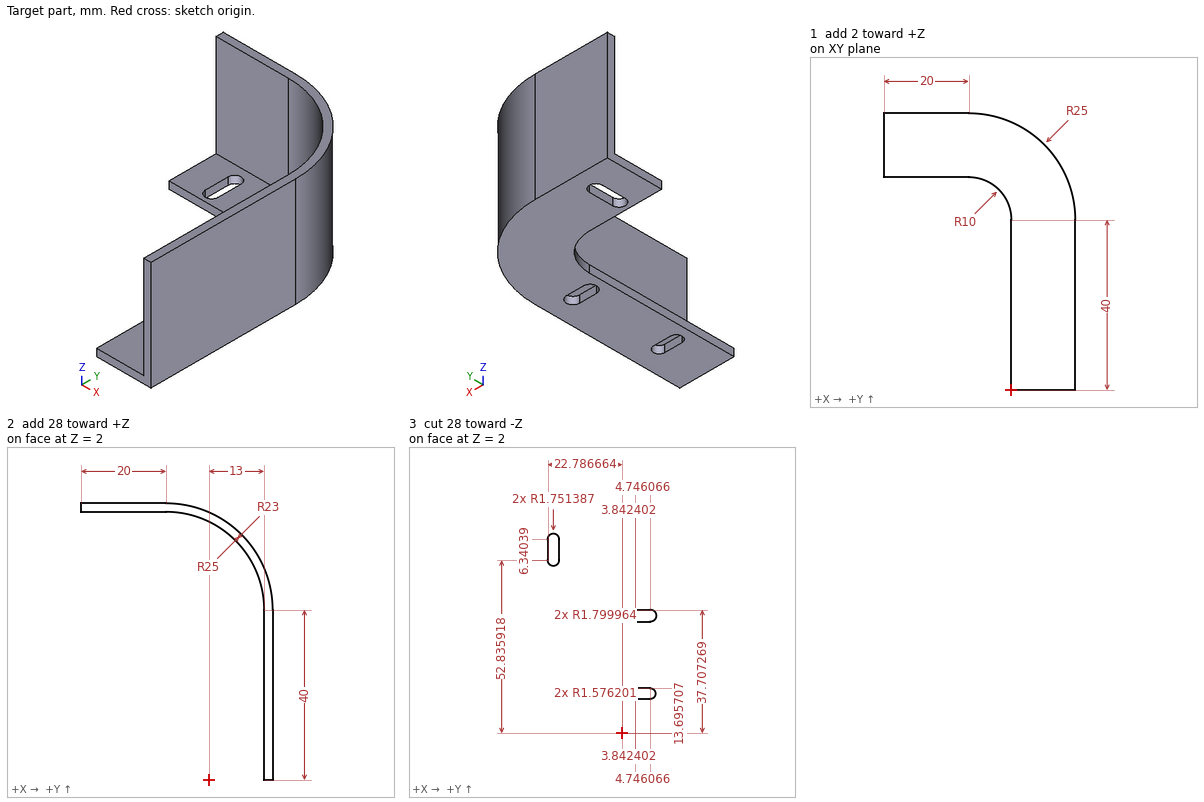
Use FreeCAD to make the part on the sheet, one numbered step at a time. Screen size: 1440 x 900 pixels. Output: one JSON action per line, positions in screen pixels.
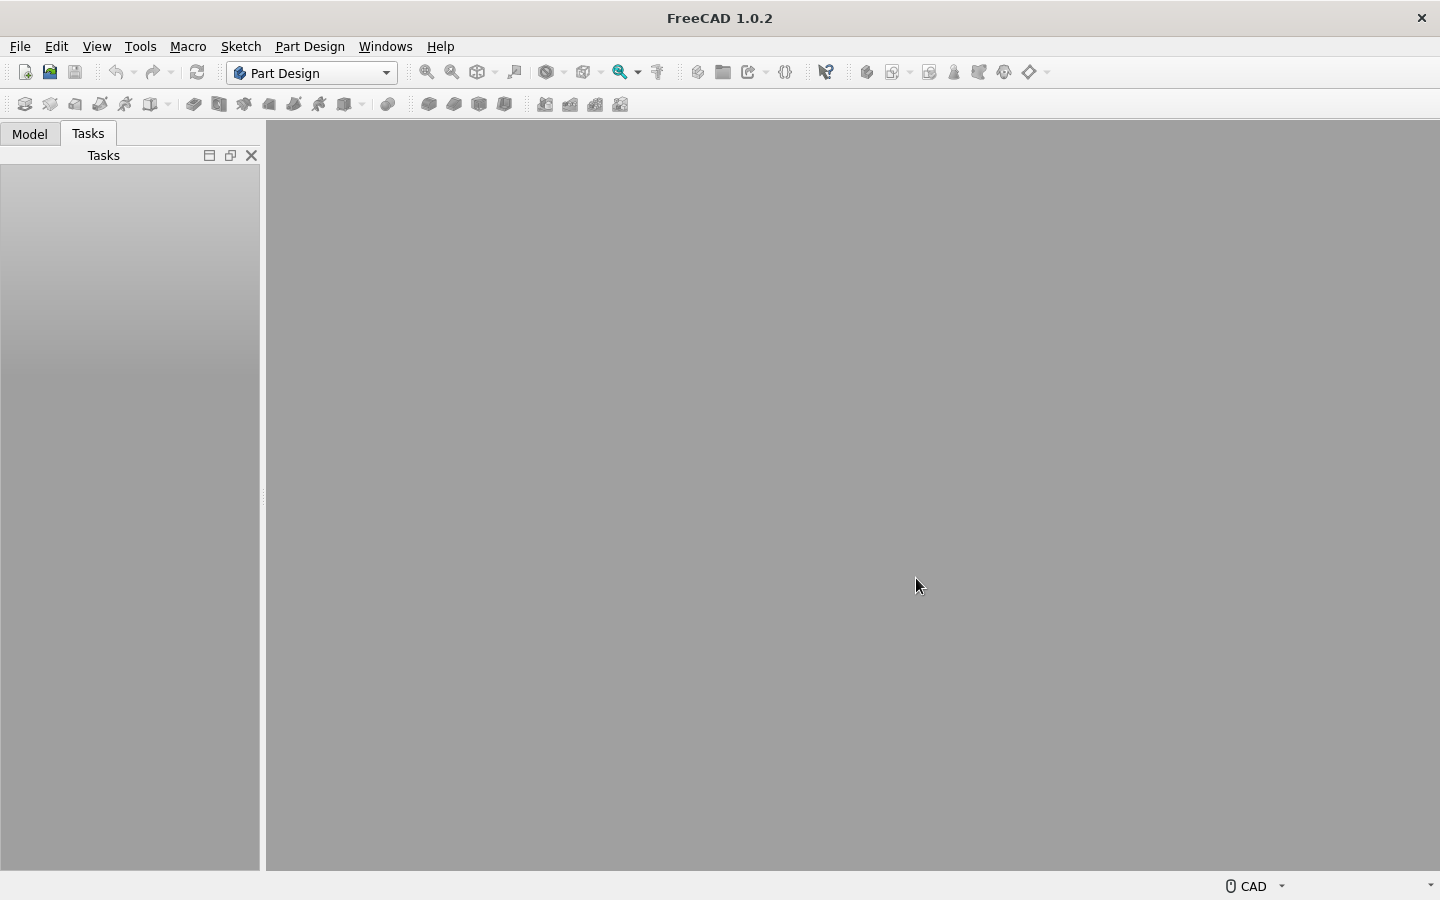
{"action": "left_click", "coordinate": [25, 72]}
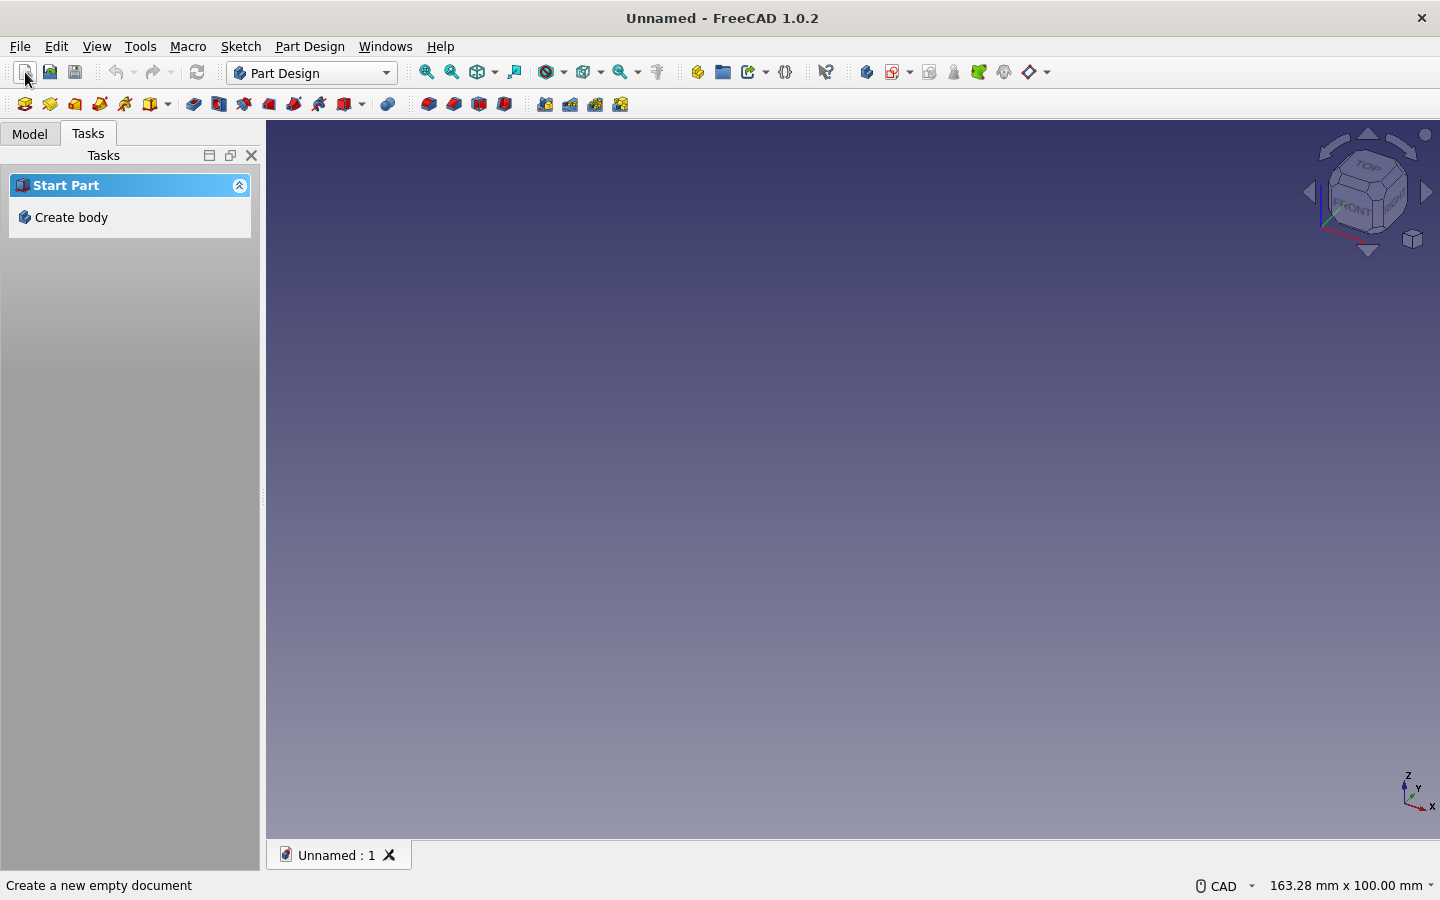
{"action": "left_click", "coordinate": [892, 72]}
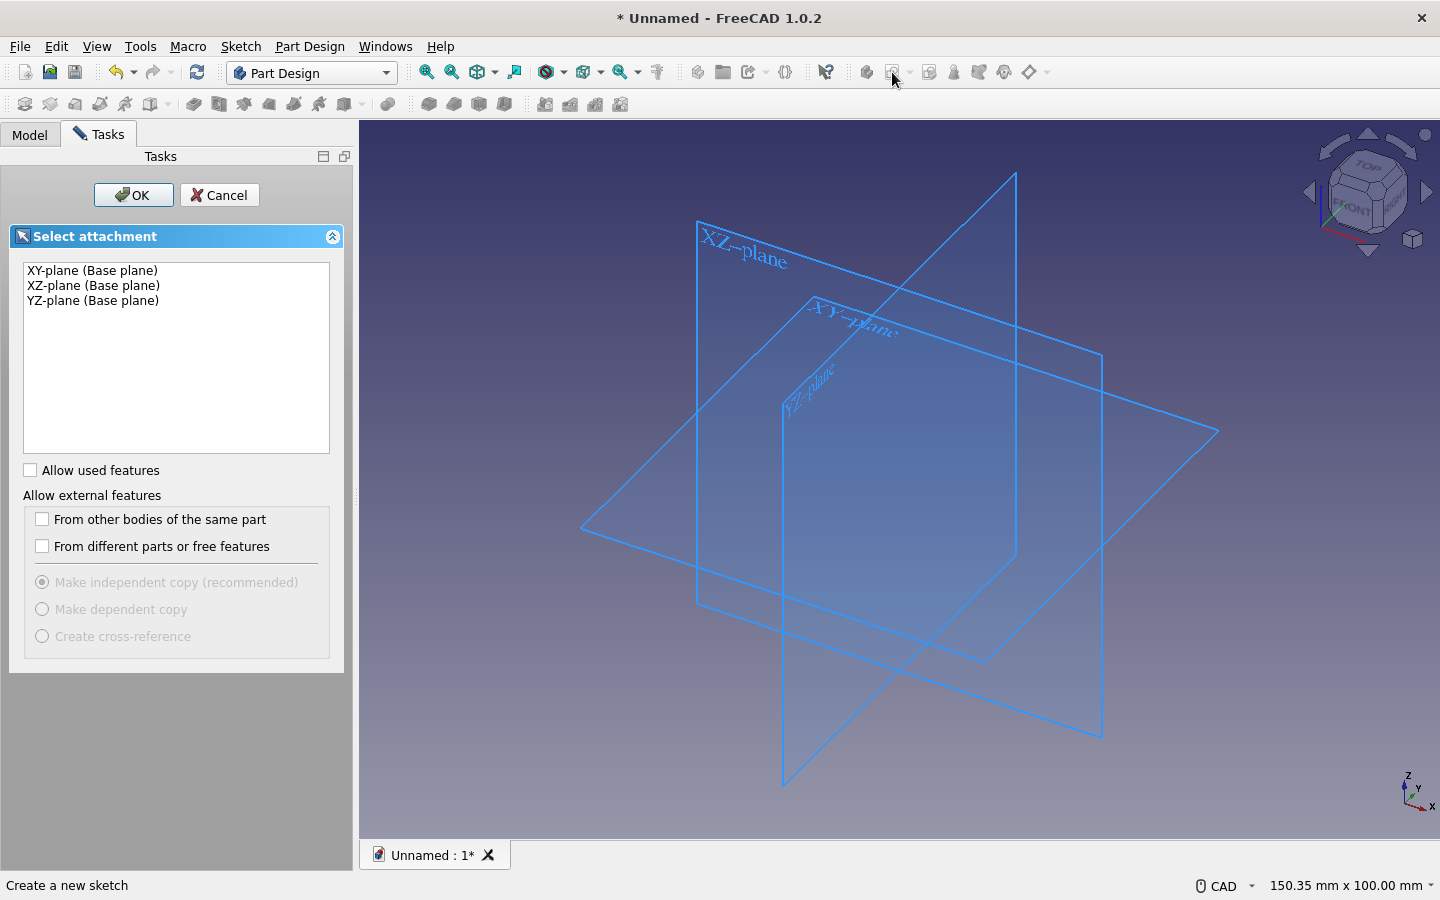
{"action": "left_click", "coordinate": [84, 270]}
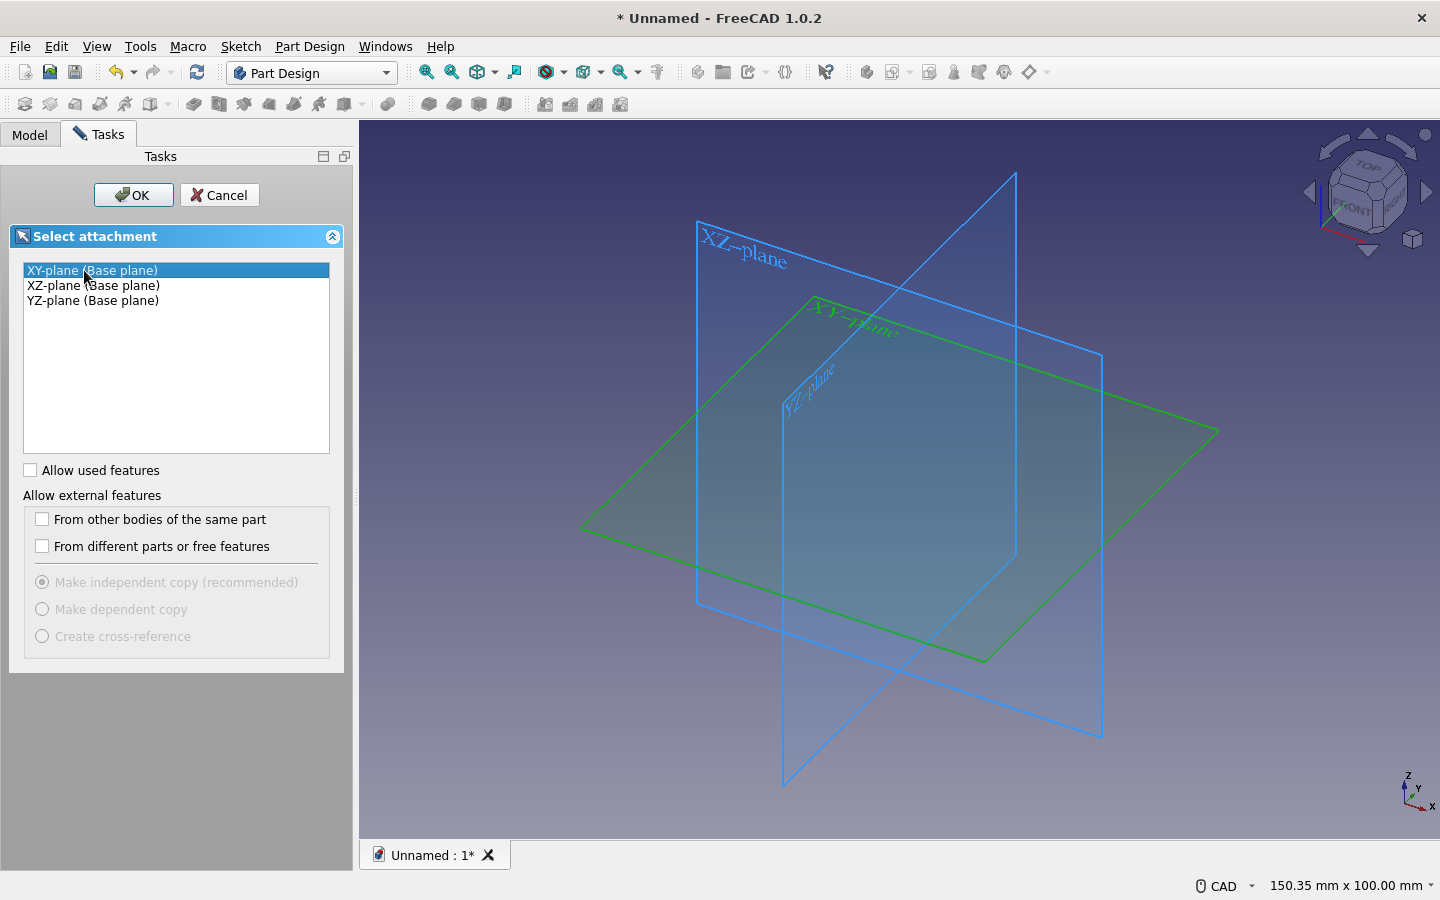
{"action": "left_click", "coordinate": [134, 195]}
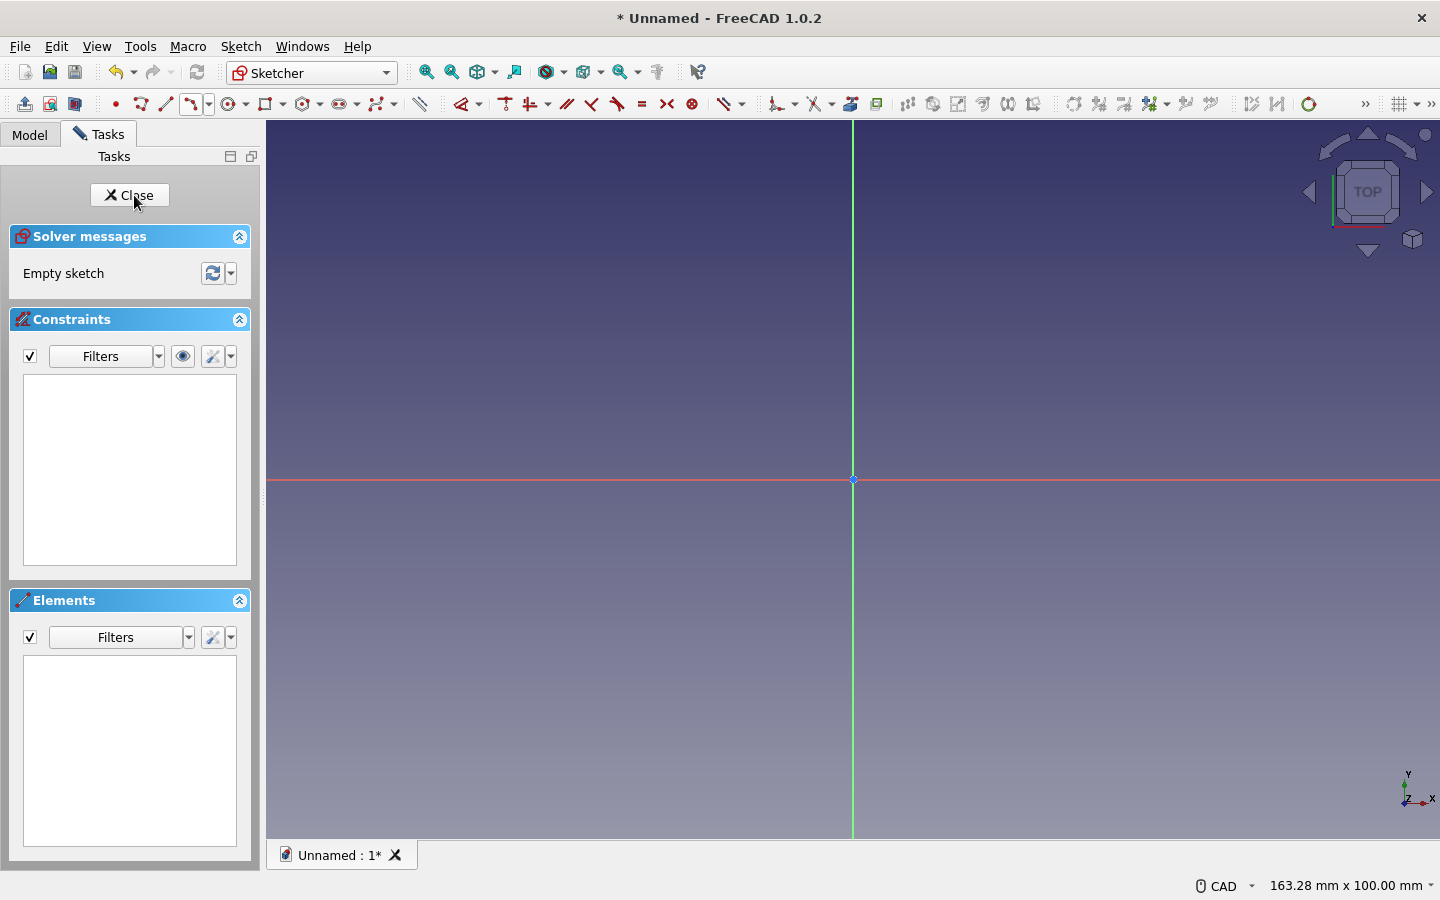
{"action": "scroll", "coordinate": [755, 811], "scroll_direction": "down", "scroll_amount": 2}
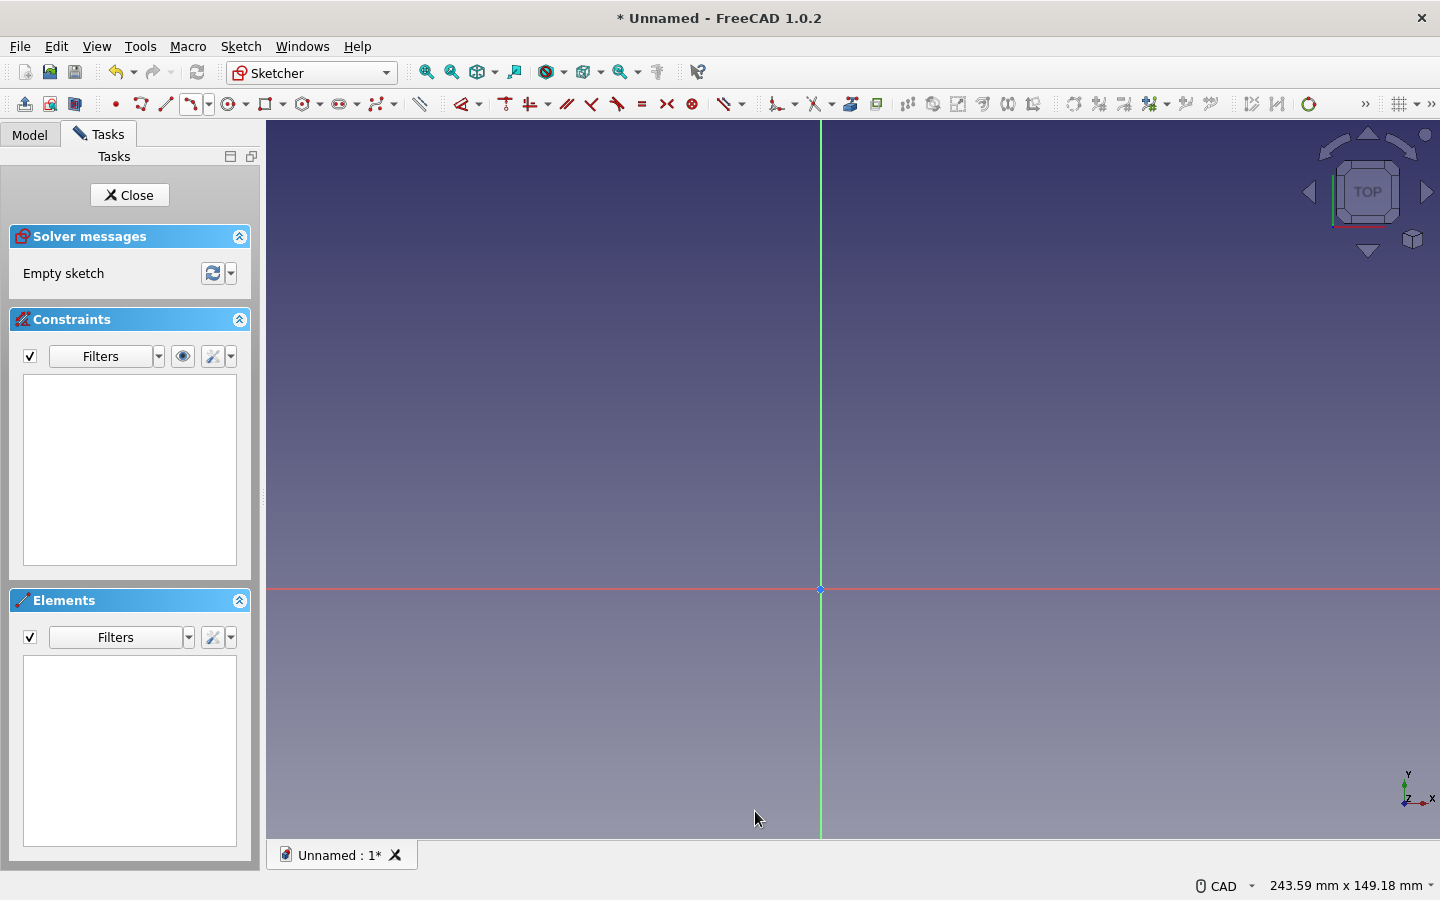
{"action": "scroll", "coordinate": [785, 337], "scroll_direction": "up", "scroll_amount": 2}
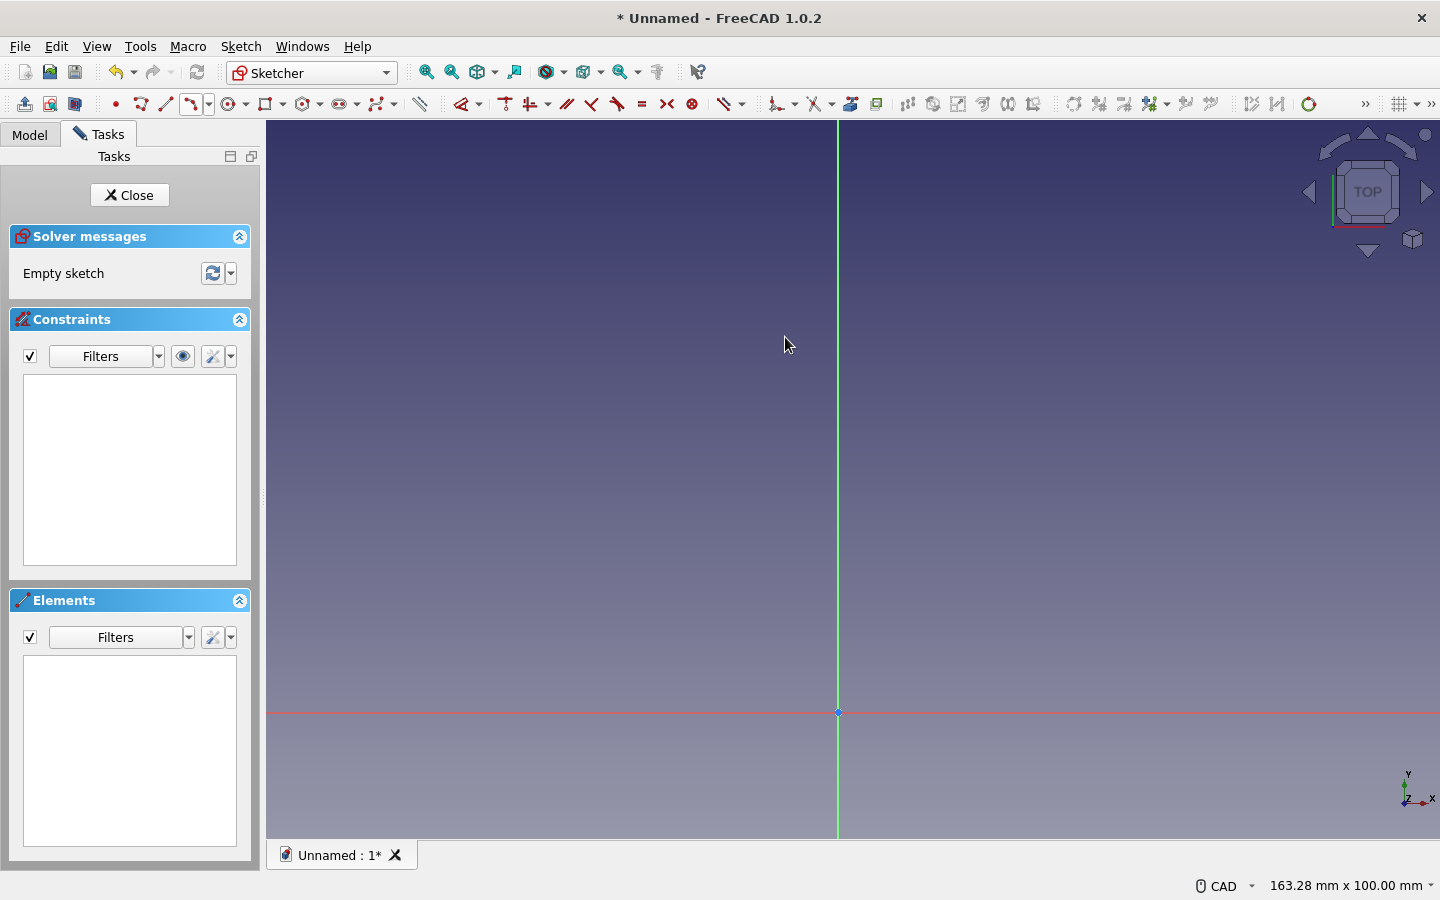
{"action": "left_click", "coordinate": [141, 104]}